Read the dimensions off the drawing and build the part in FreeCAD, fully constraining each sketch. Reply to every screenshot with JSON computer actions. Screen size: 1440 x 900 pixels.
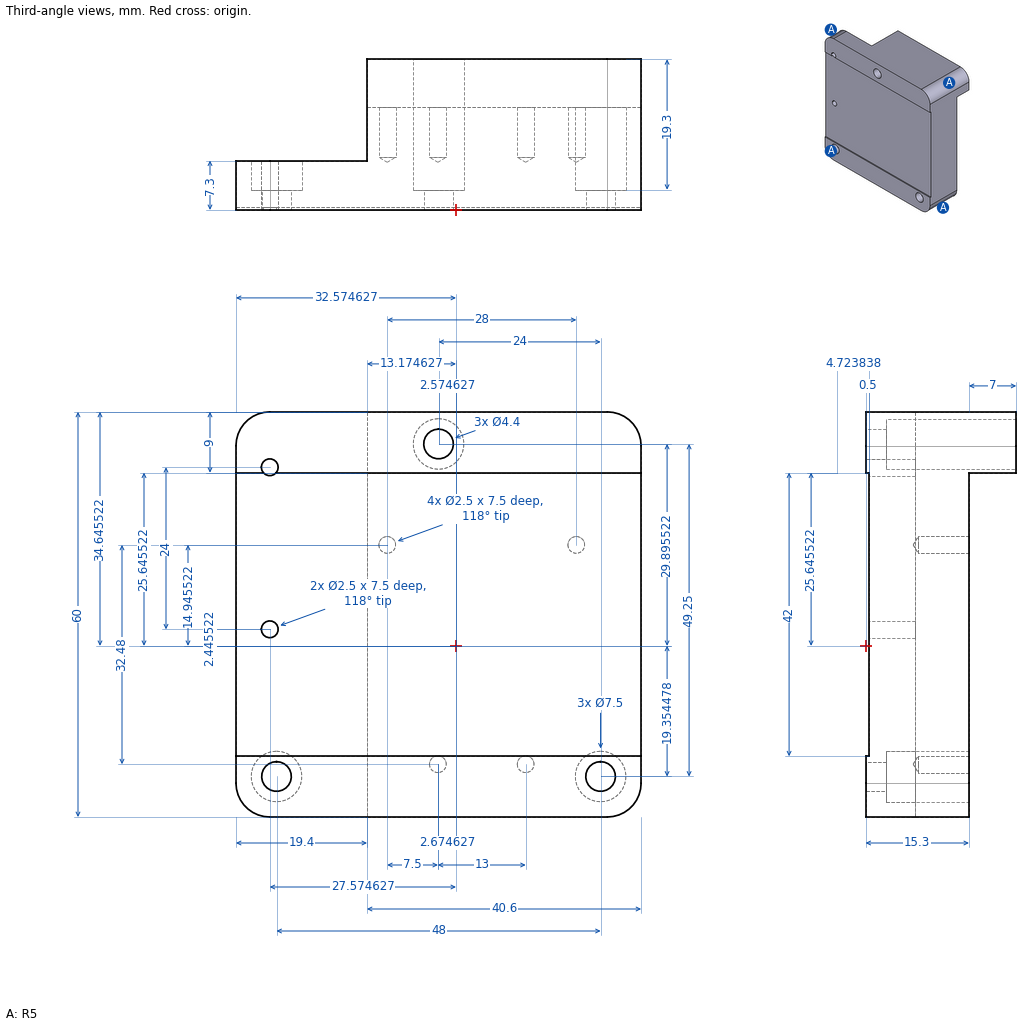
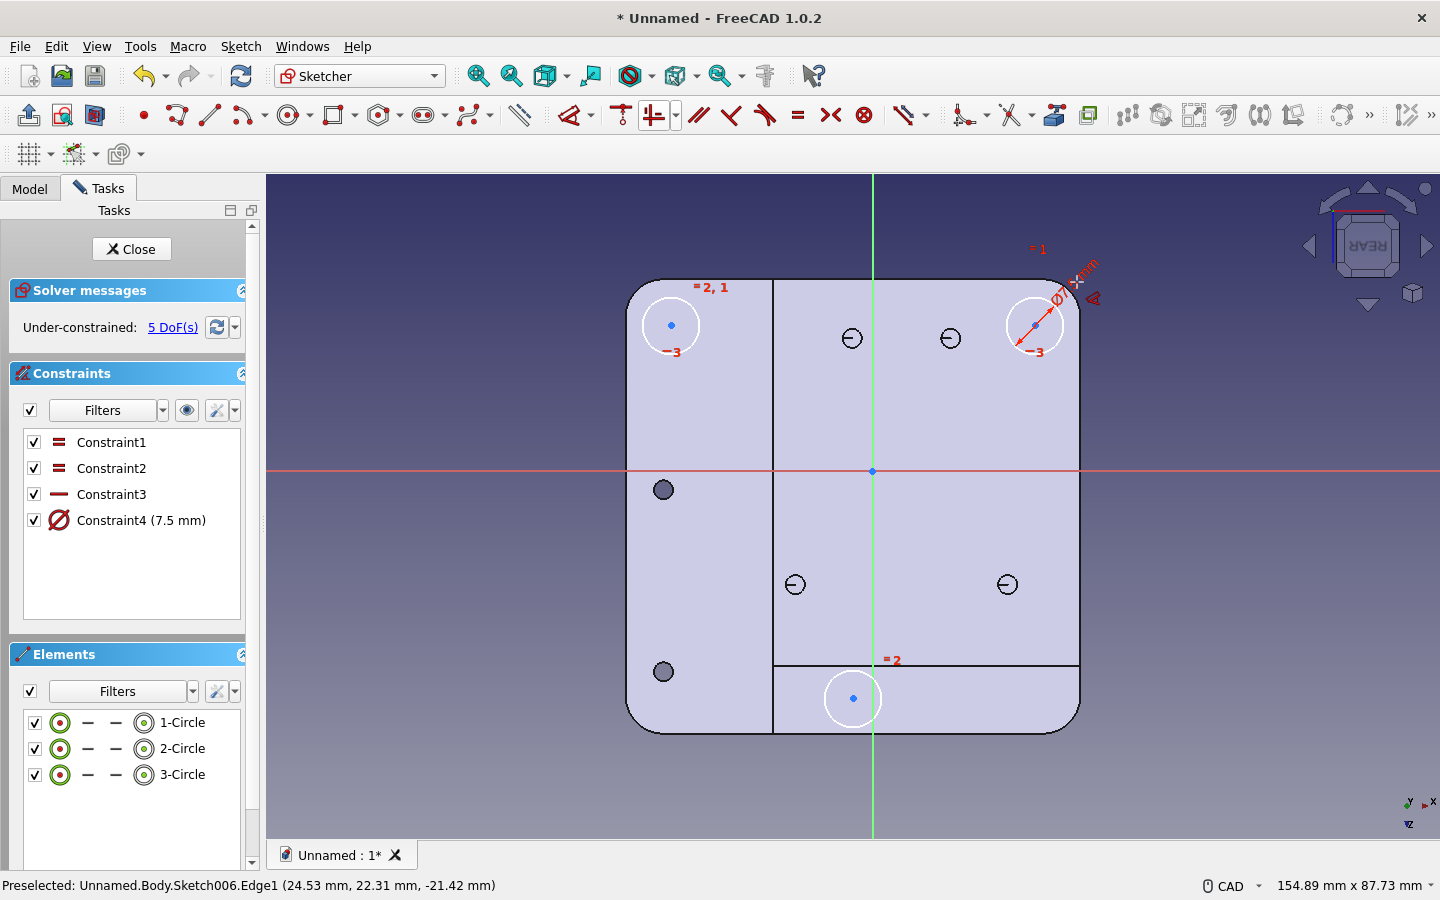
{"action": "left_click", "coordinate": [1035, 326]}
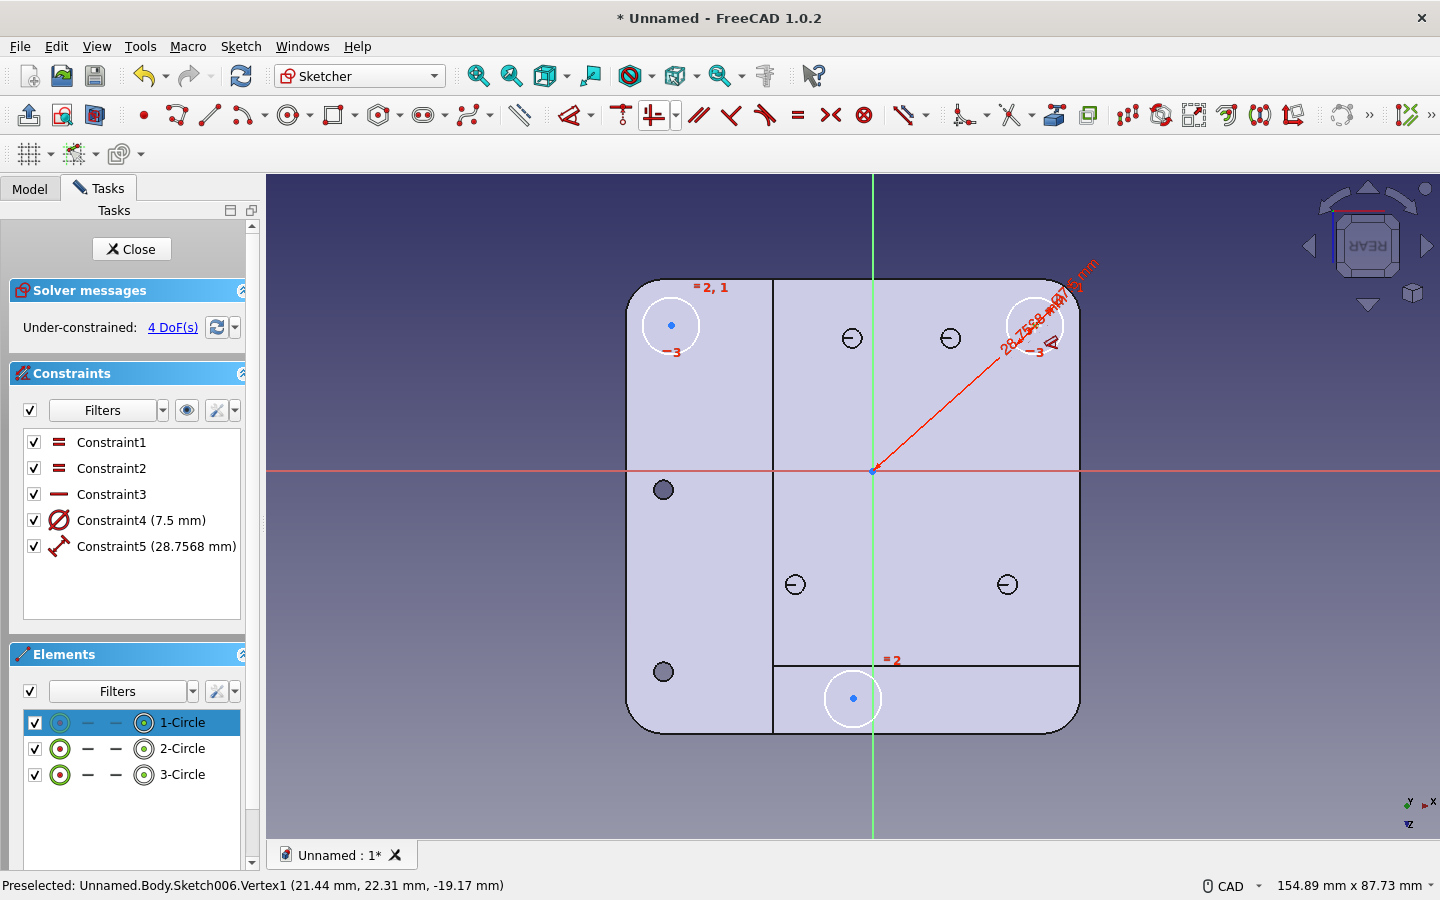
{"action": "left_click", "coordinate": [671, 326]}
{"action": "left_click", "coordinate": [853, 292]}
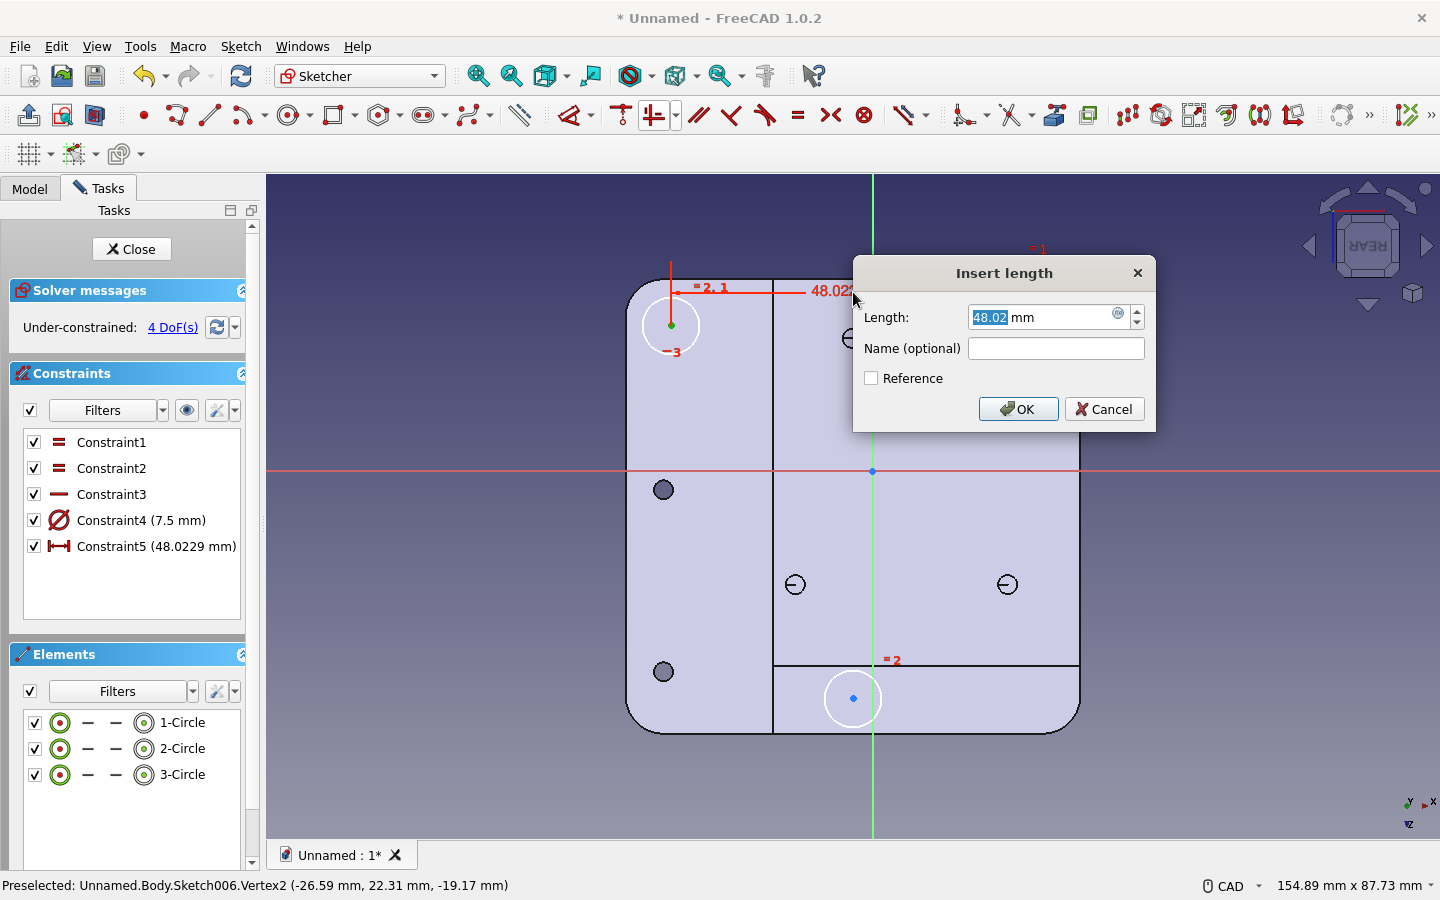
{"action": "type", "text": "48"}
{"action": "key", "text": "Return"}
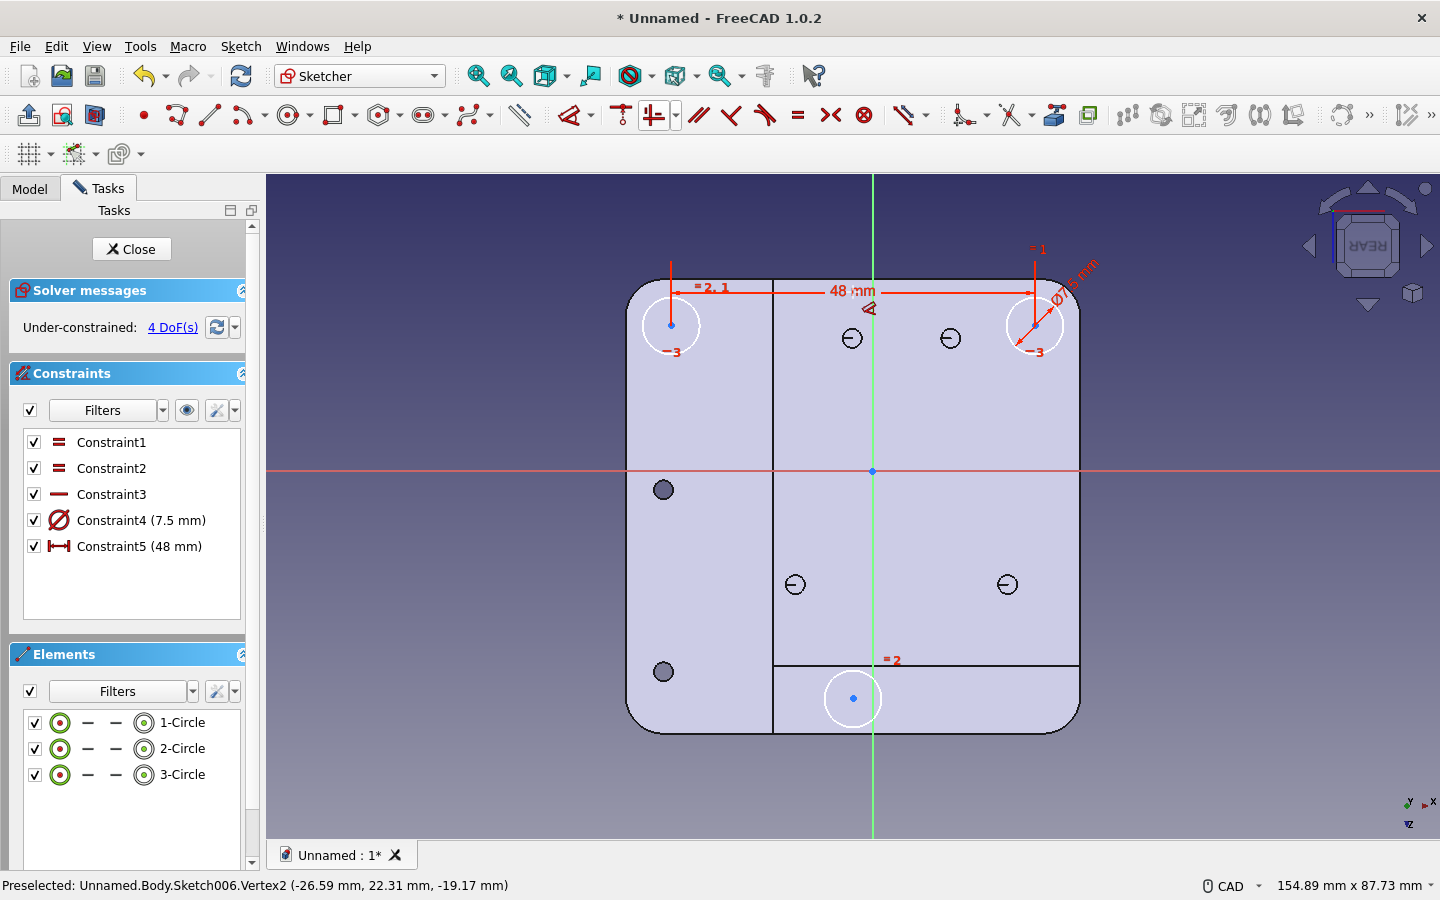
{"action": "left_click", "coordinate": [1035, 326]}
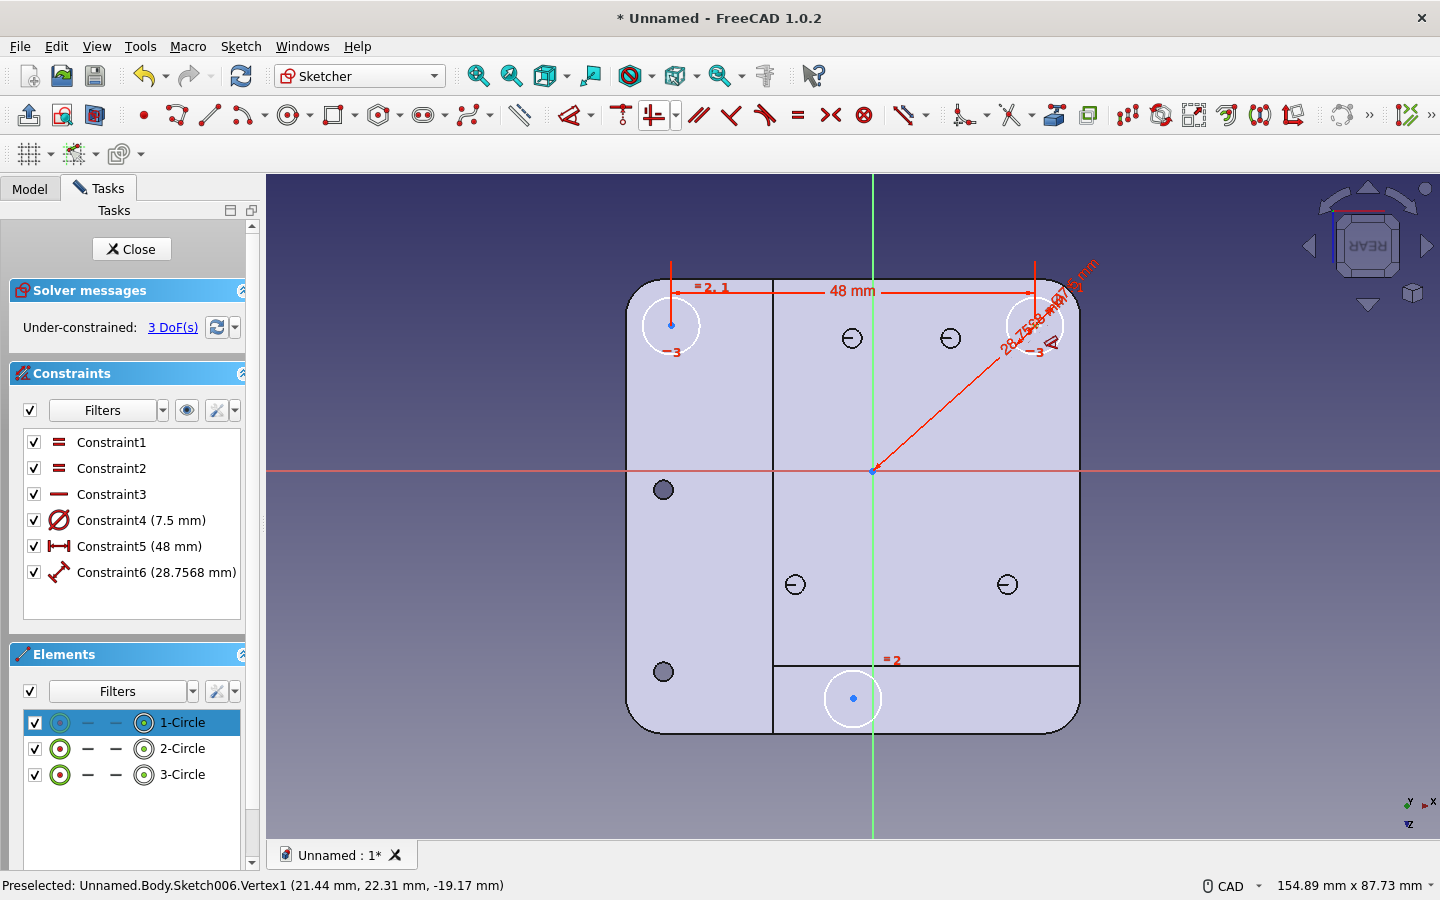
{"action": "left_click", "coordinate": [853, 699]}
{"action": "left_click", "coordinate": [944, 733]}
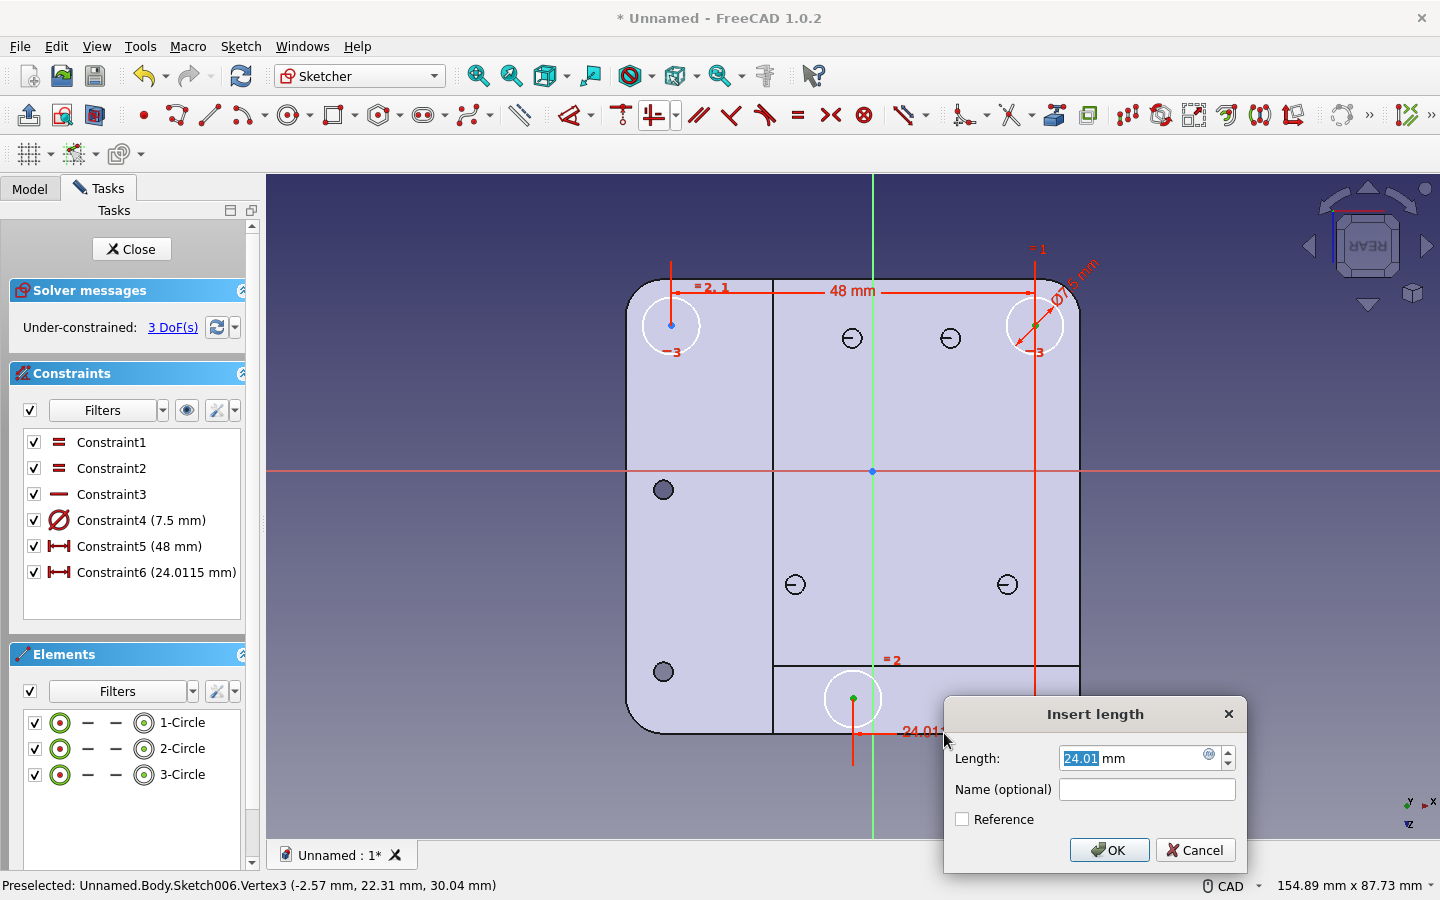
{"action": "type", "text": "24"}
{"action": "key", "text": "Return"}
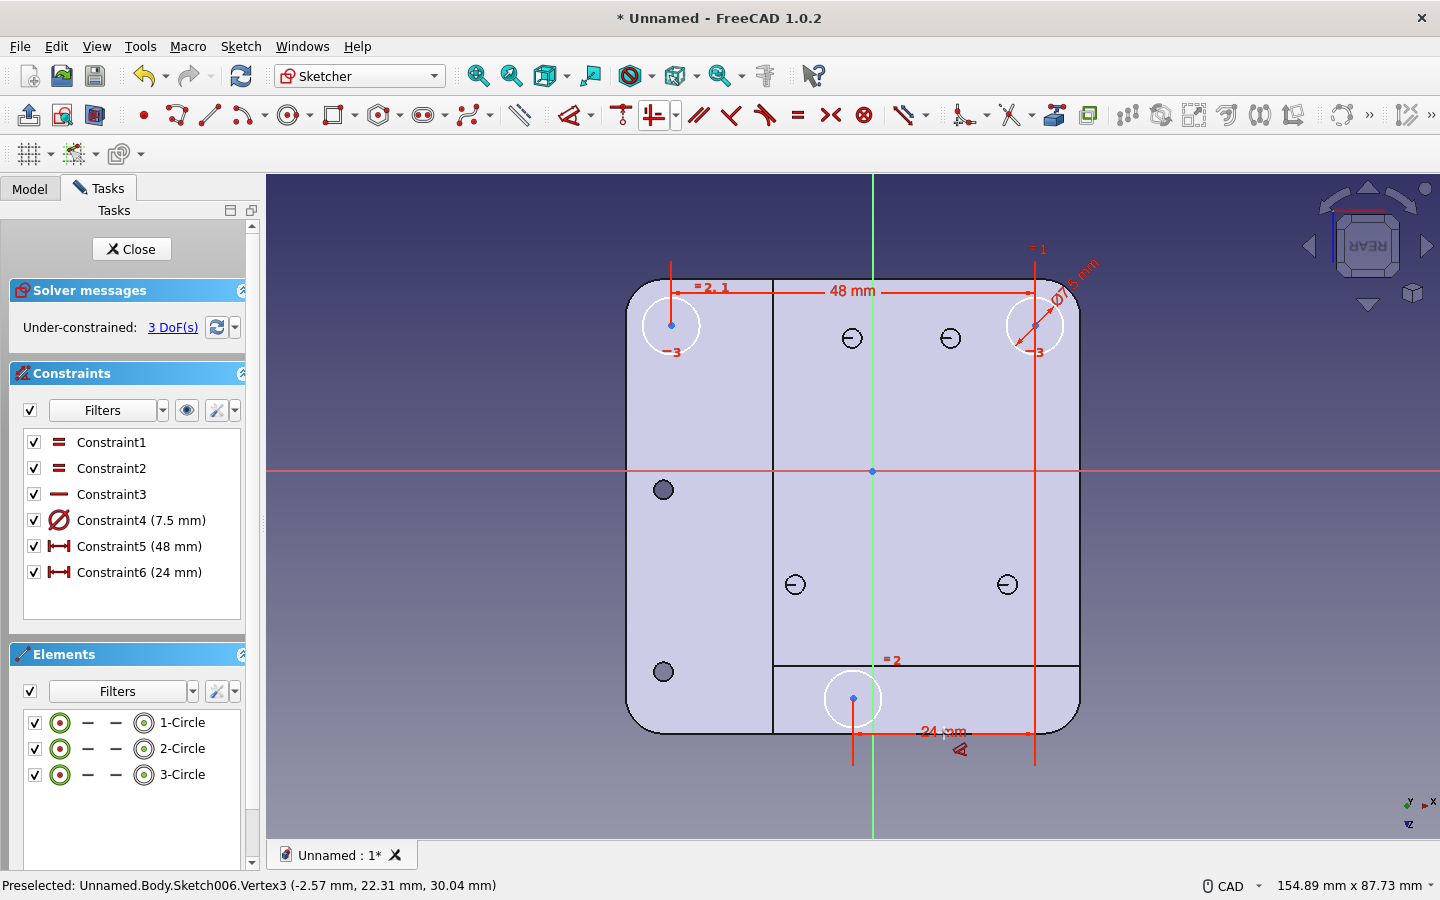
{"action": "left_click", "coordinate": [1035, 326]}